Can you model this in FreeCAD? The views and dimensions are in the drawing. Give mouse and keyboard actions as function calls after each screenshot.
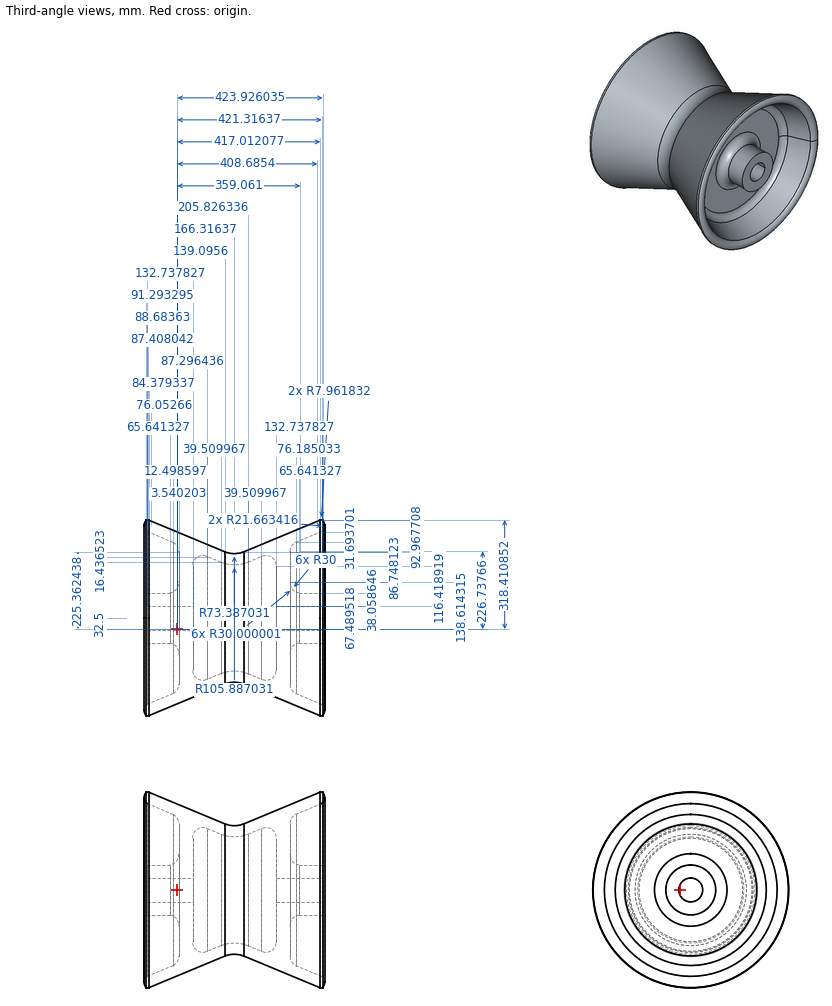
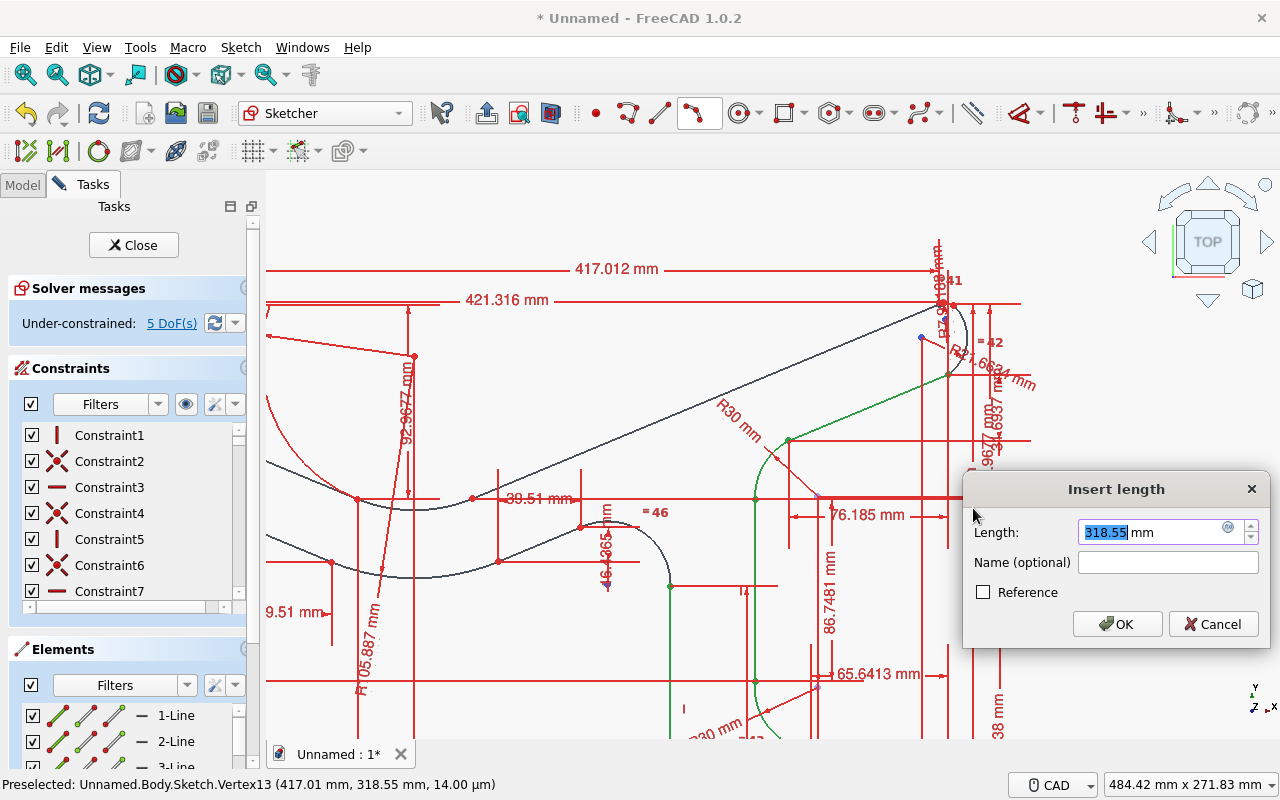
text(318.410852)
key(Return)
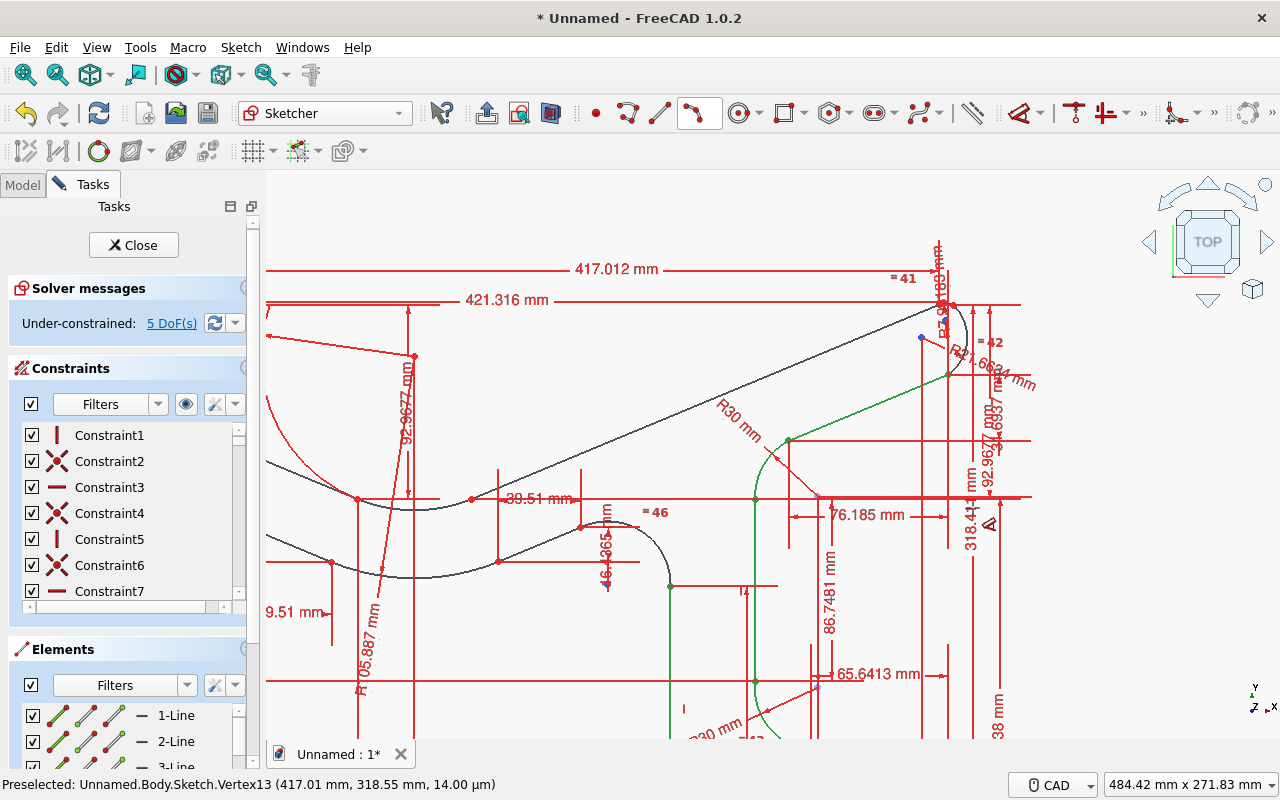
scroll(941, 305, down, 4)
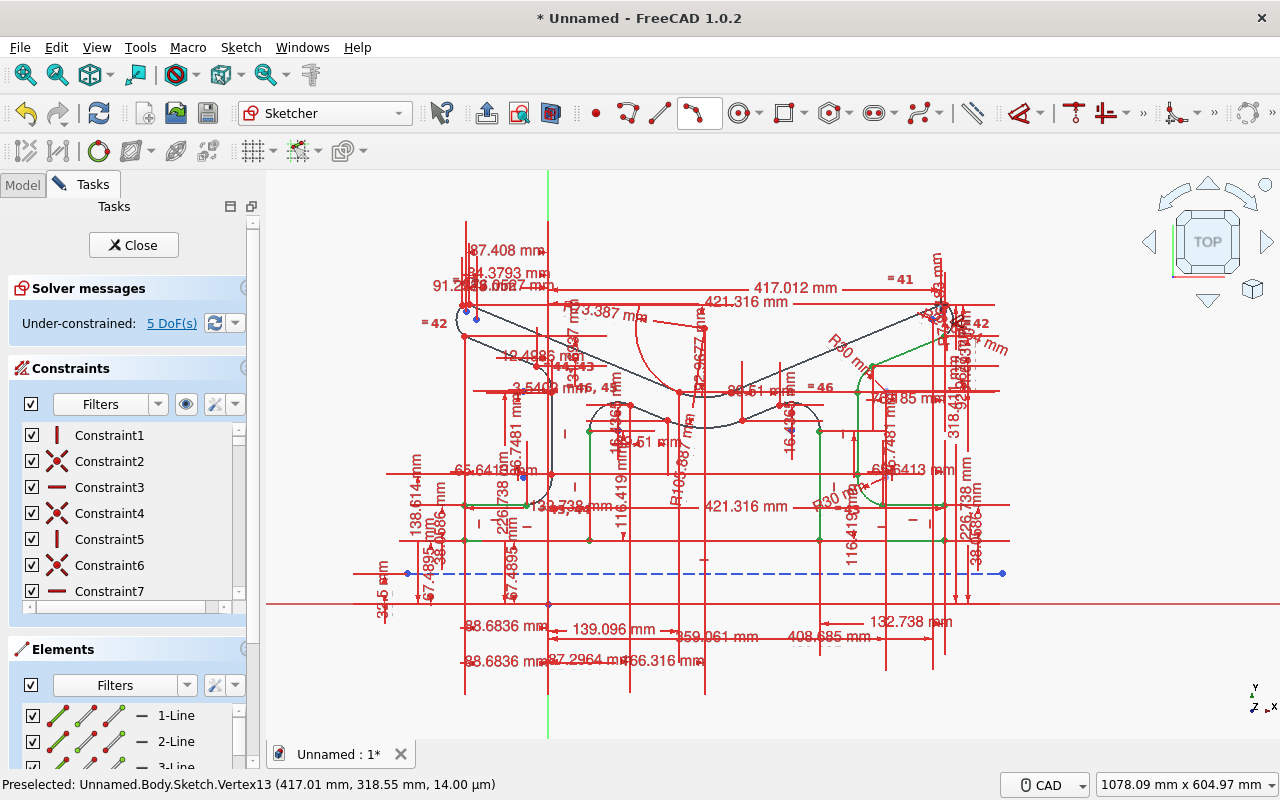
click(552, 393)
click(610, 547)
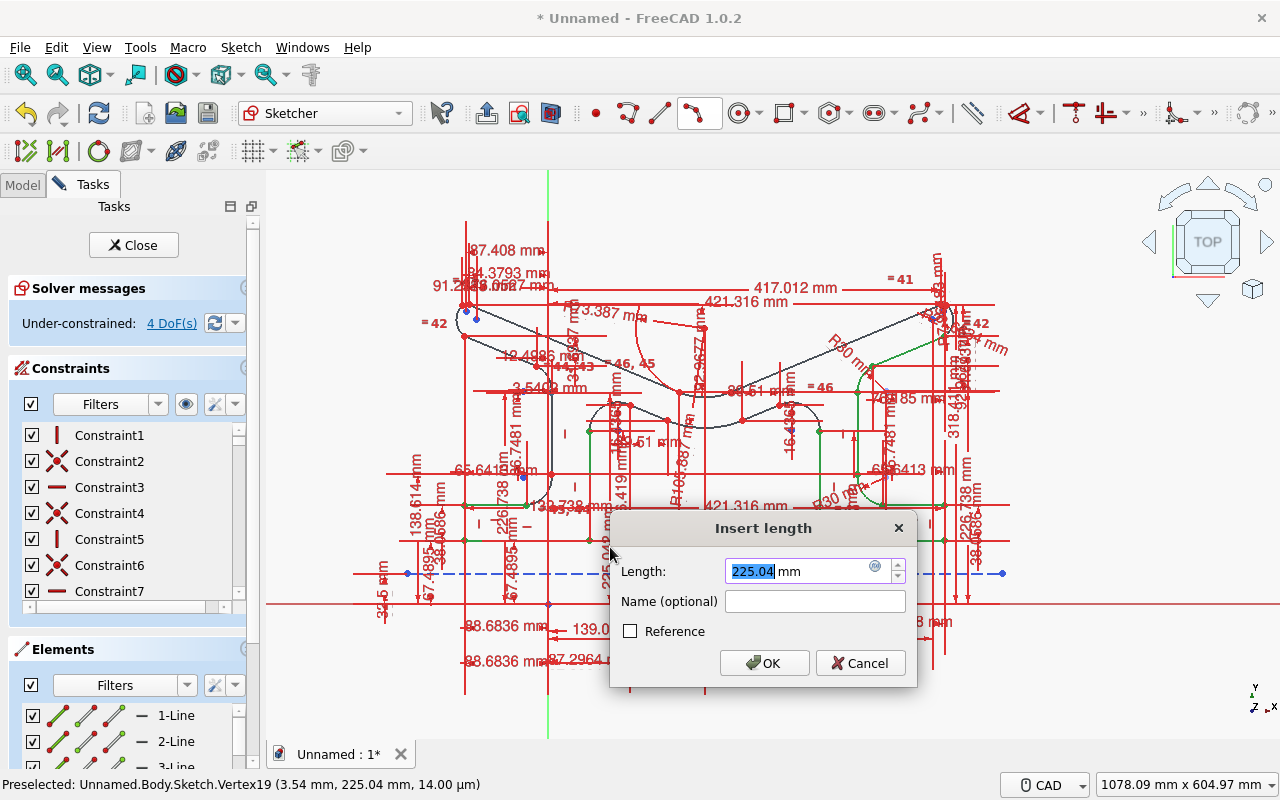
text(225.362438)
key(Return)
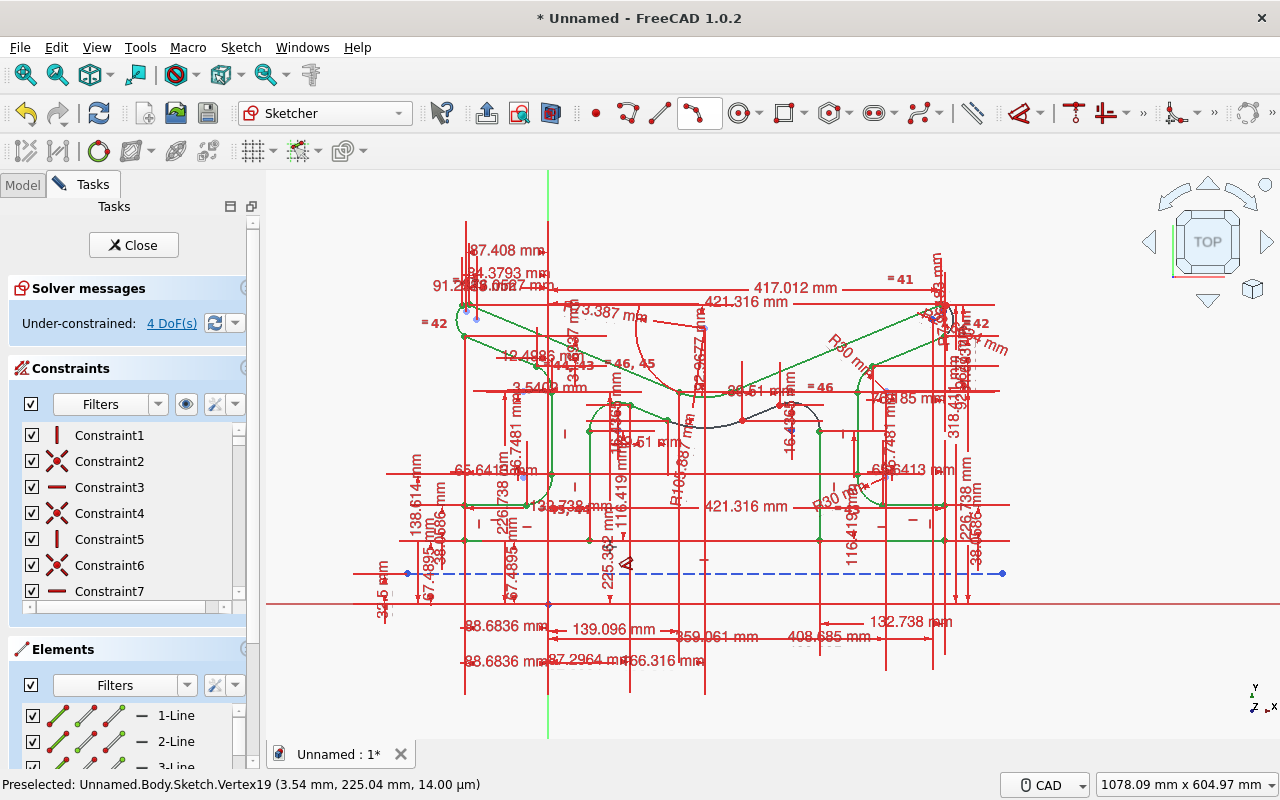
click(742, 421)
click(645, 686)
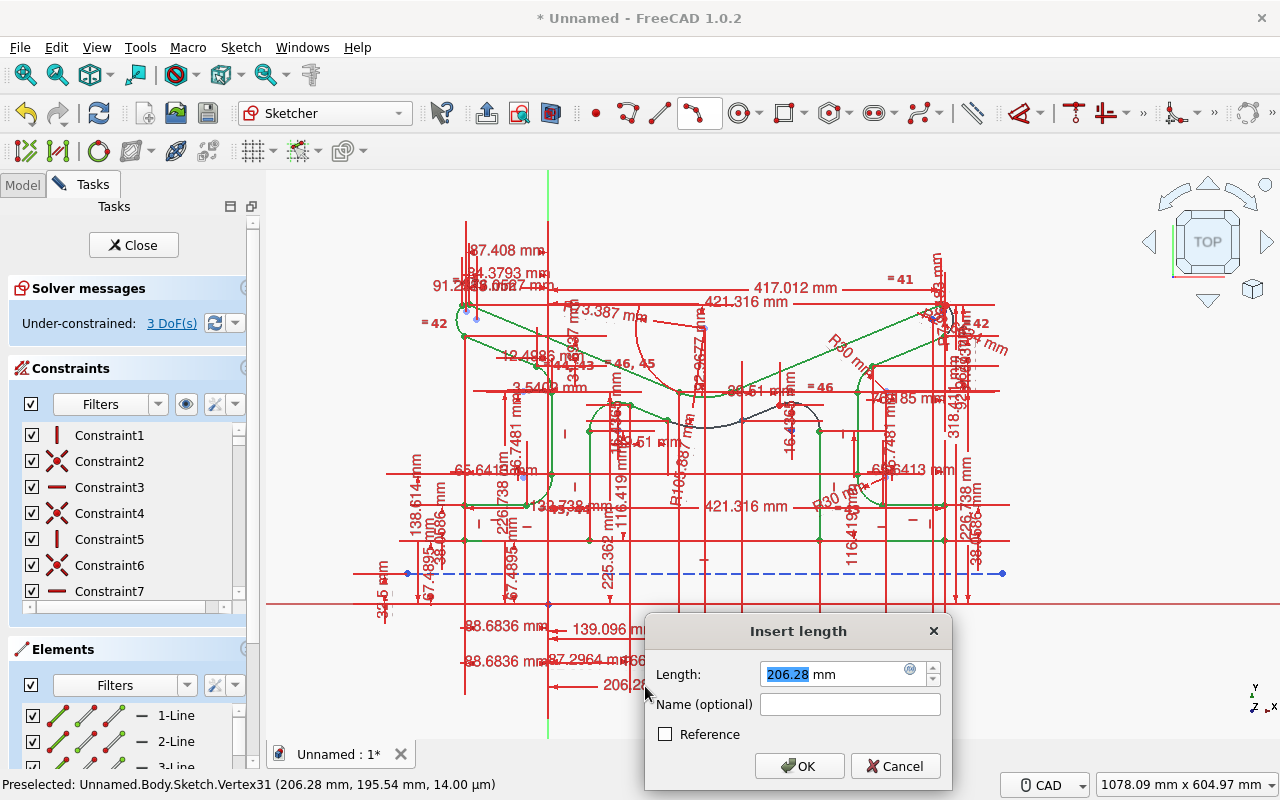
text(205.826336)
key(Return)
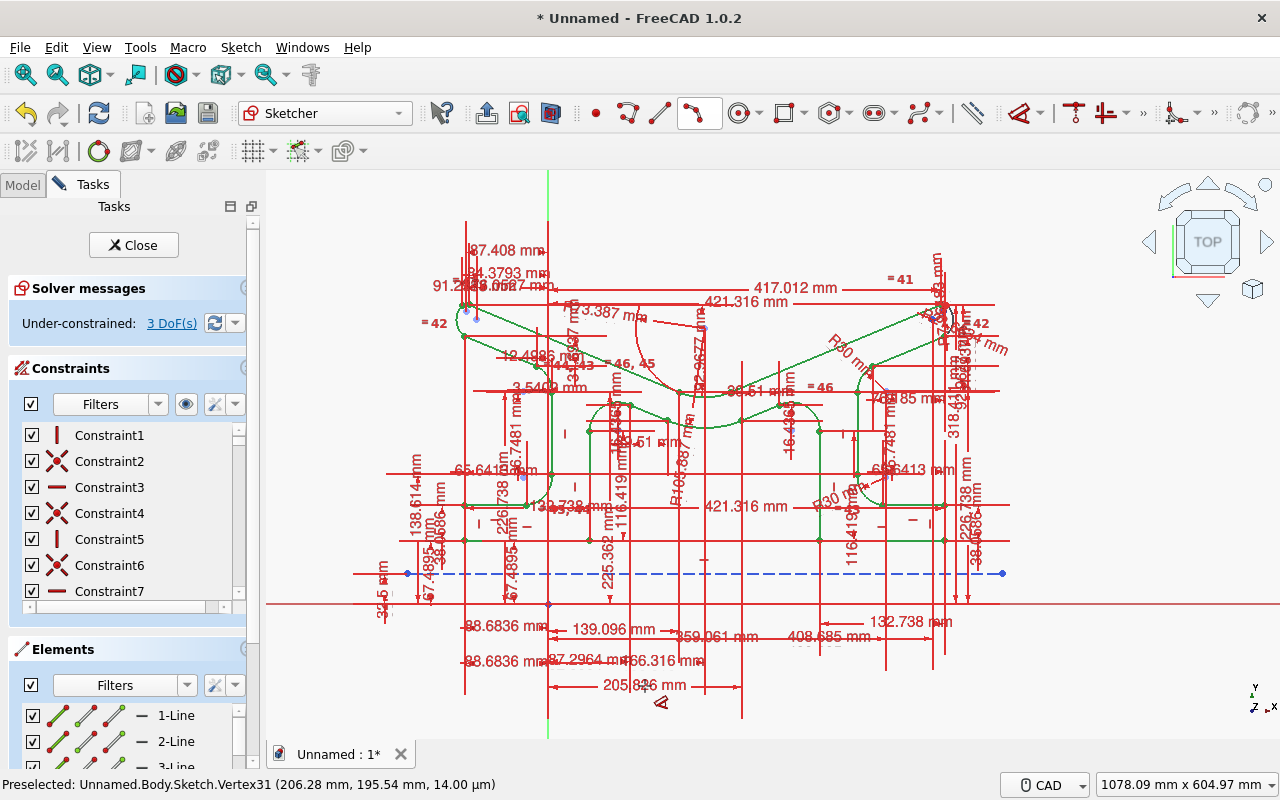
scroll(947, 305, up, 4)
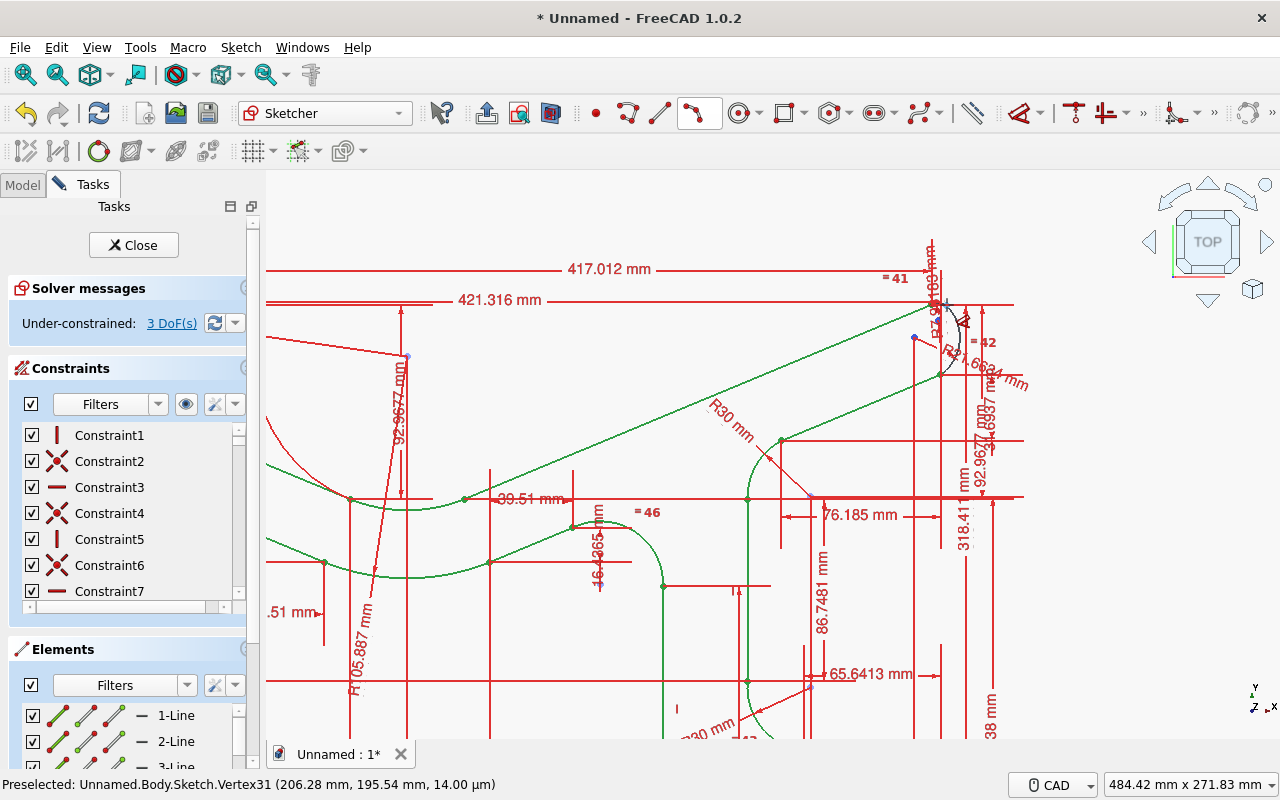
click(946, 305)
click(470, 271)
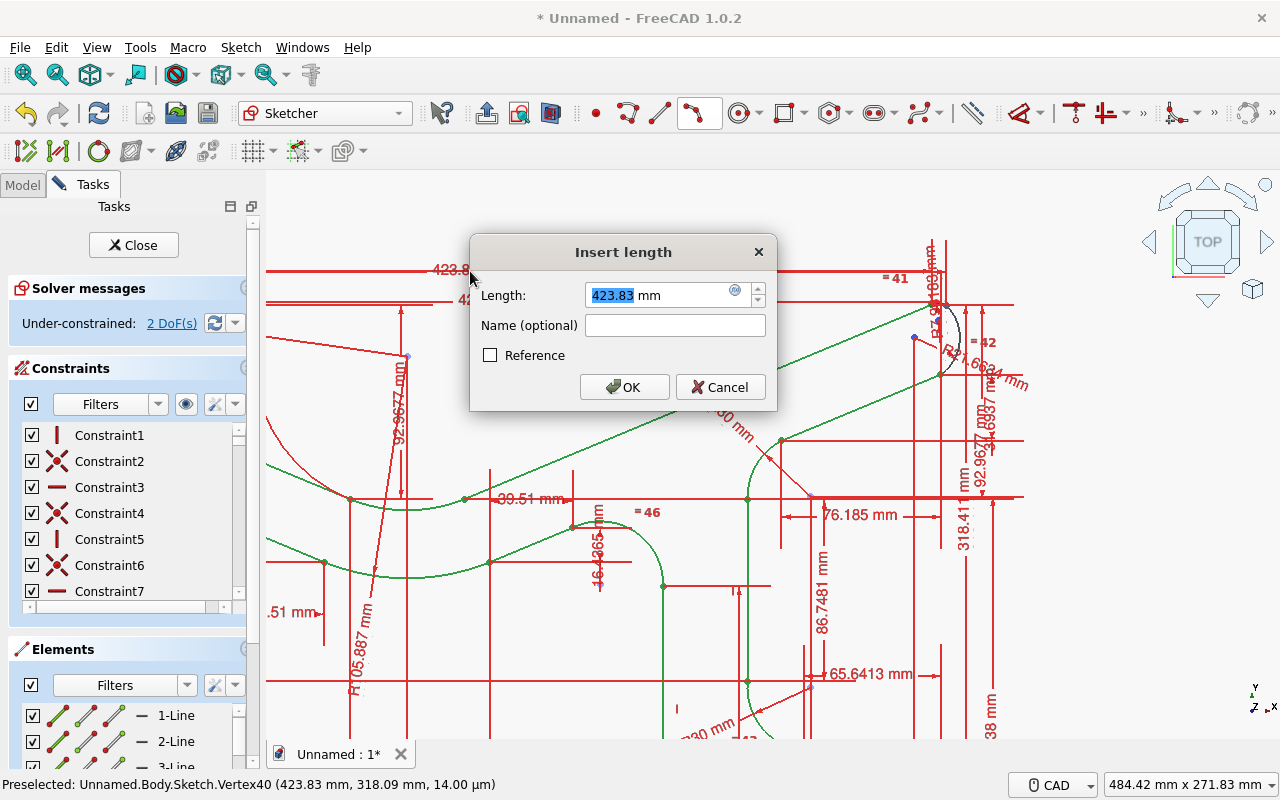
text(423.926035)
key(Return)
key(Escape)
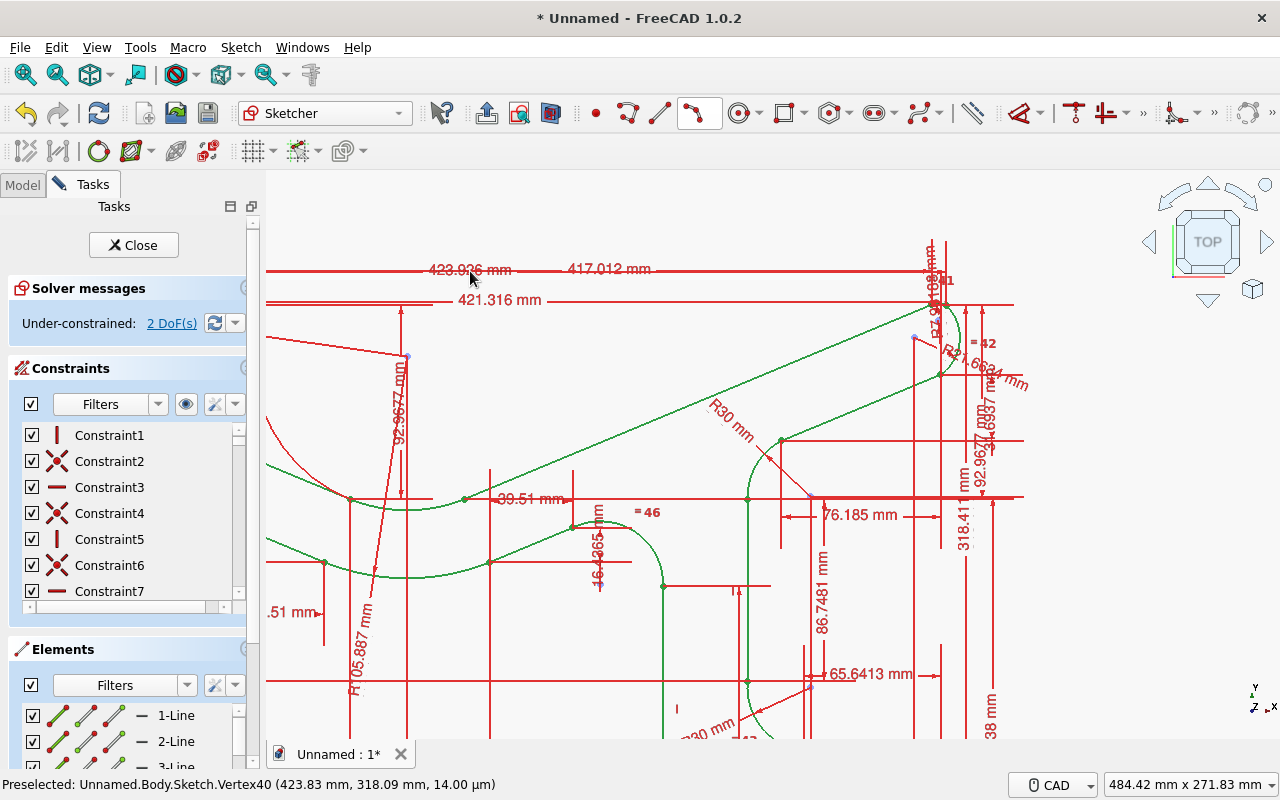
click(134, 245)